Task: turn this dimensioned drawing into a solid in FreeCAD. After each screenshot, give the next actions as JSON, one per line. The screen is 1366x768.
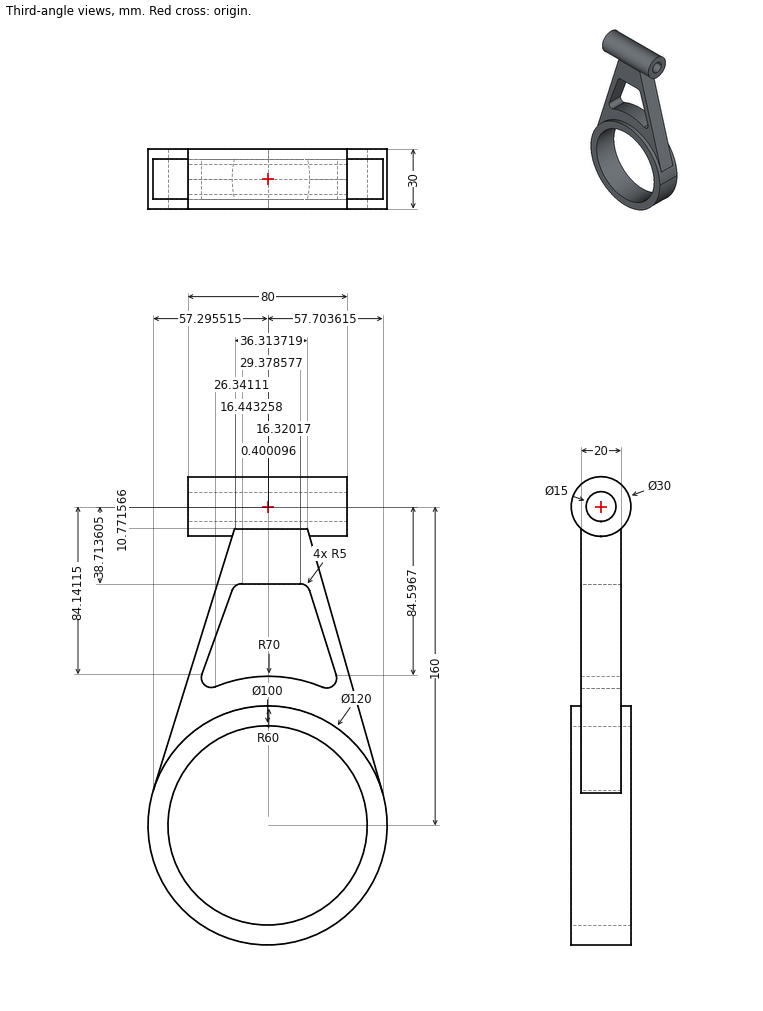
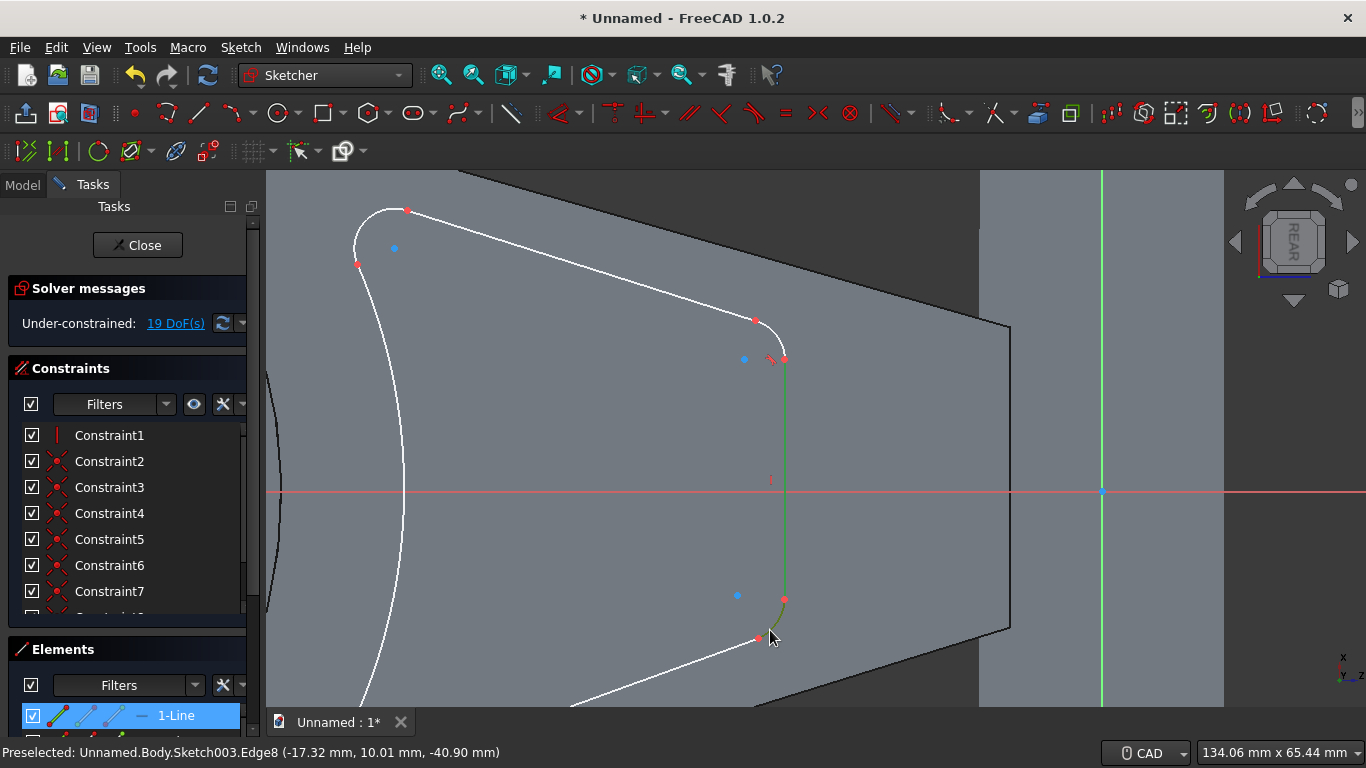
{"action": "left_click", "coordinate": [754, 114]}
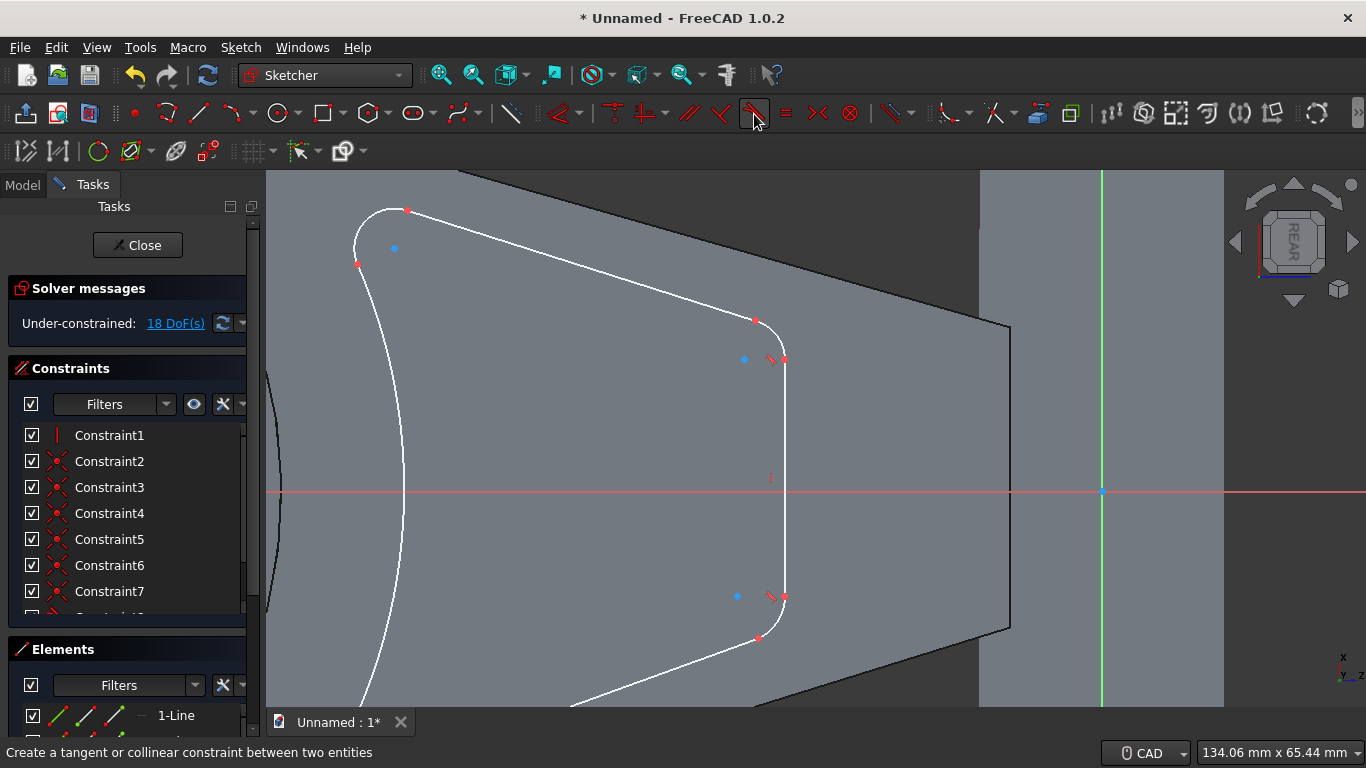
{"action": "left_click", "coordinate": [651, 288]}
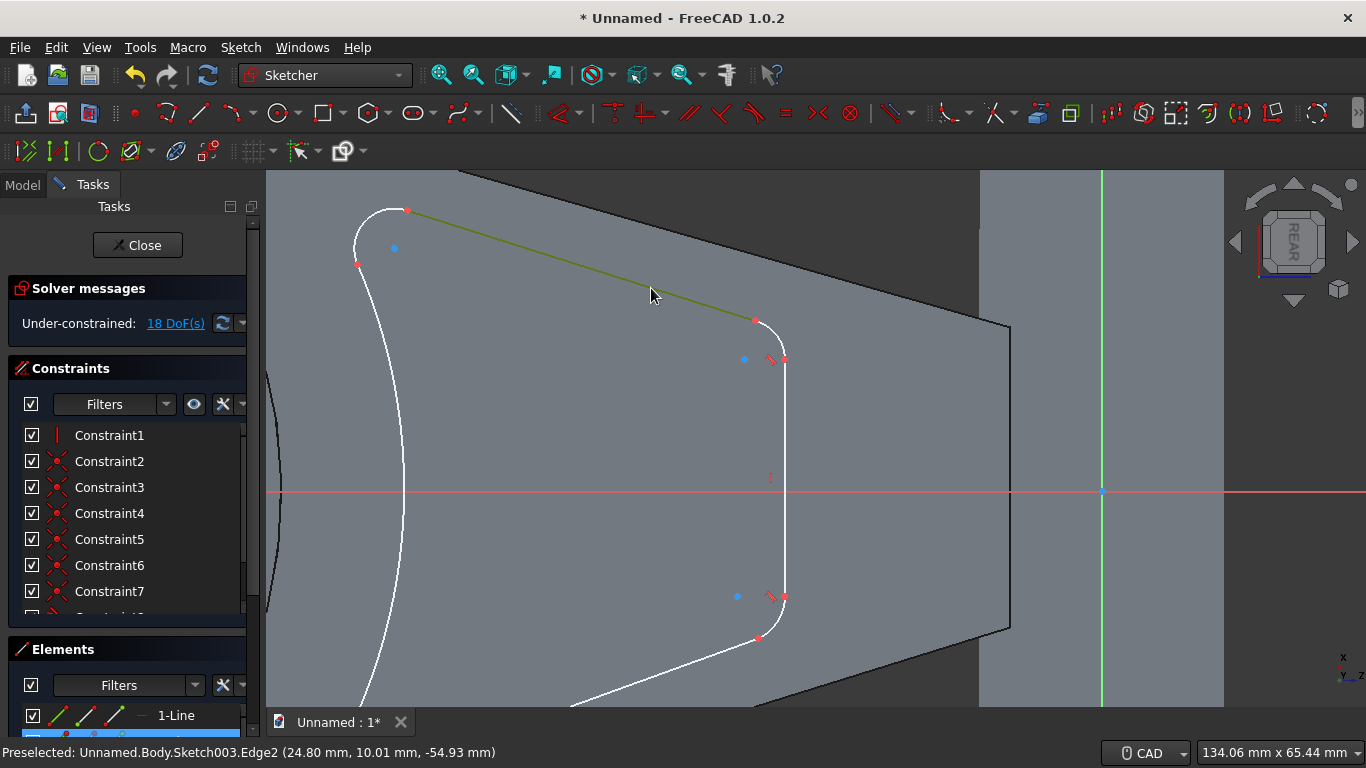
{"action": "left_click", "coordinate": [782, 344]}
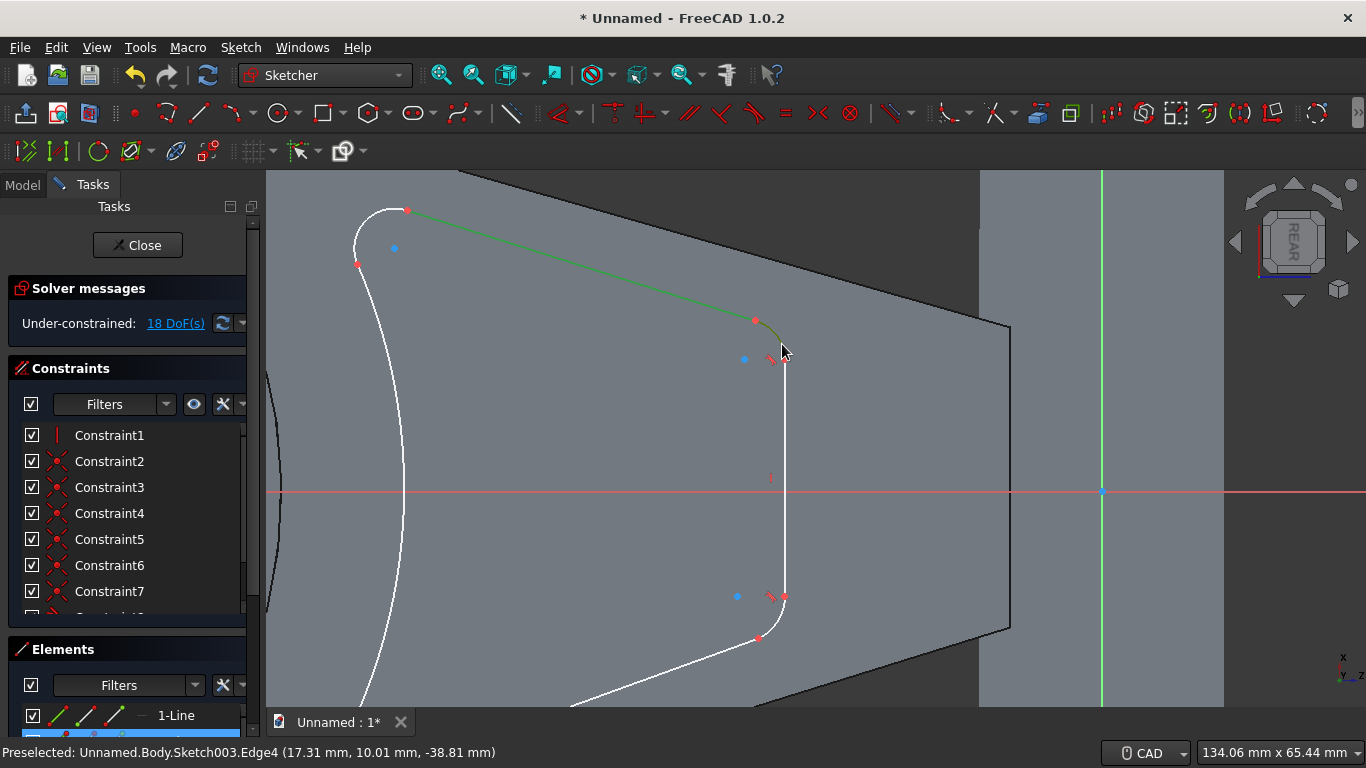
{"action": "left_click", "coordinate": [754, 114]}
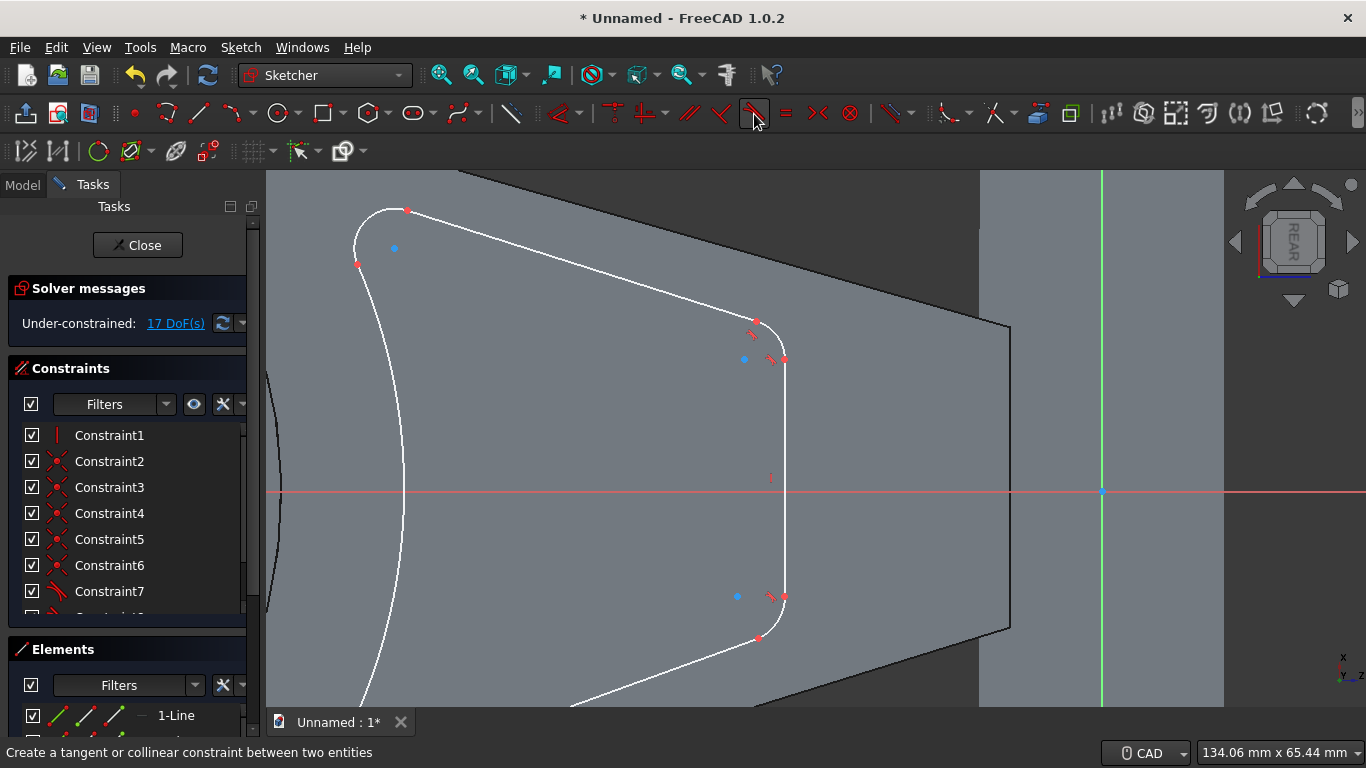
{"action": "left_click", "coordinate": [652, 288]}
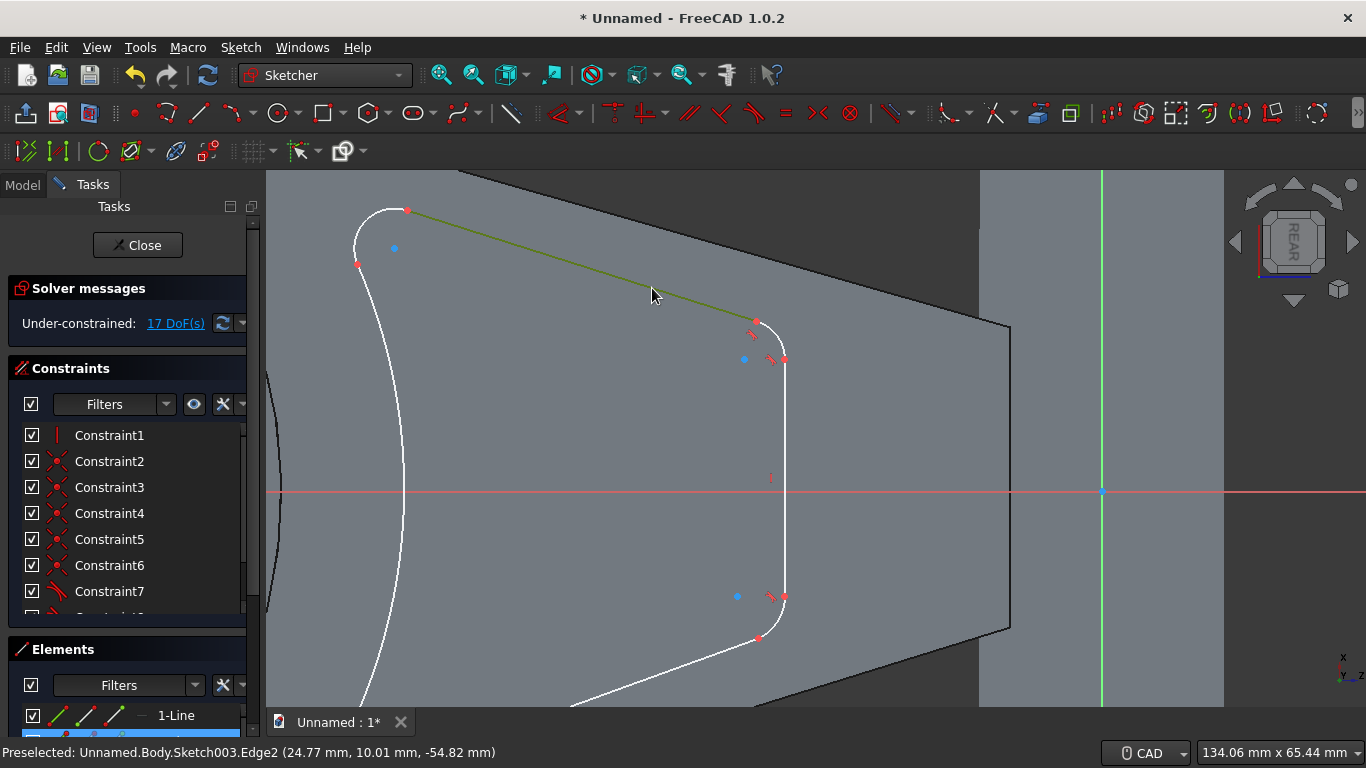
{"action": "left_click", "coordinate": [380, 211]}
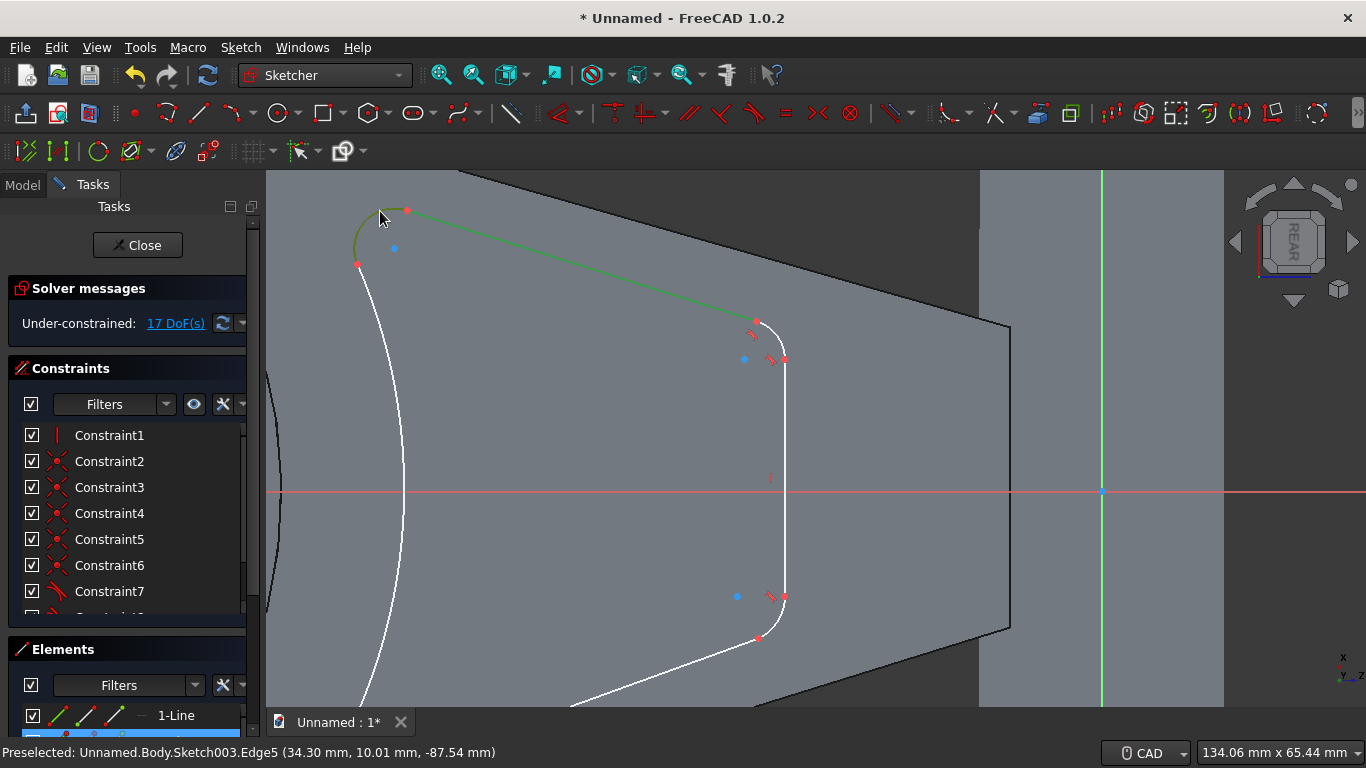
{"action": "left_click", "coordinate": [754, 114]}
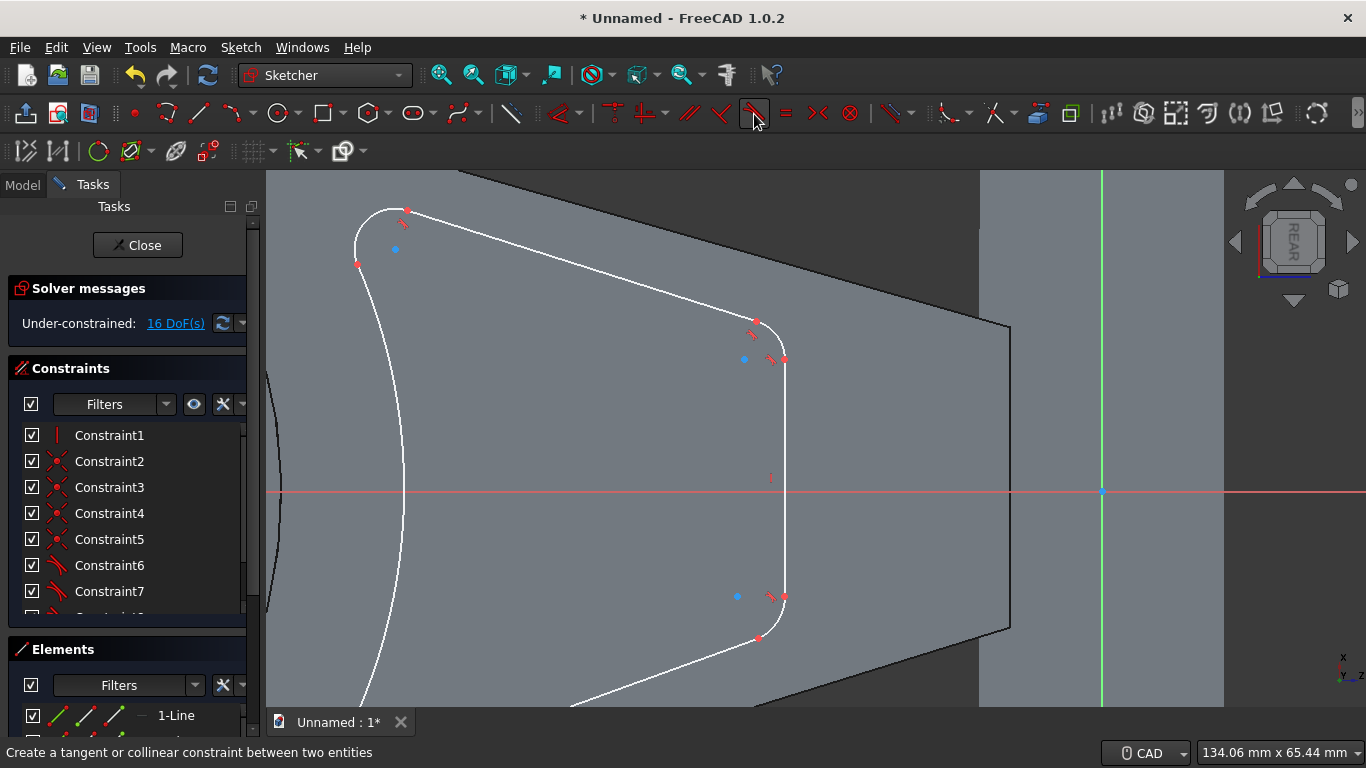
{"action": "left_click", "coordinate": [654, 676]}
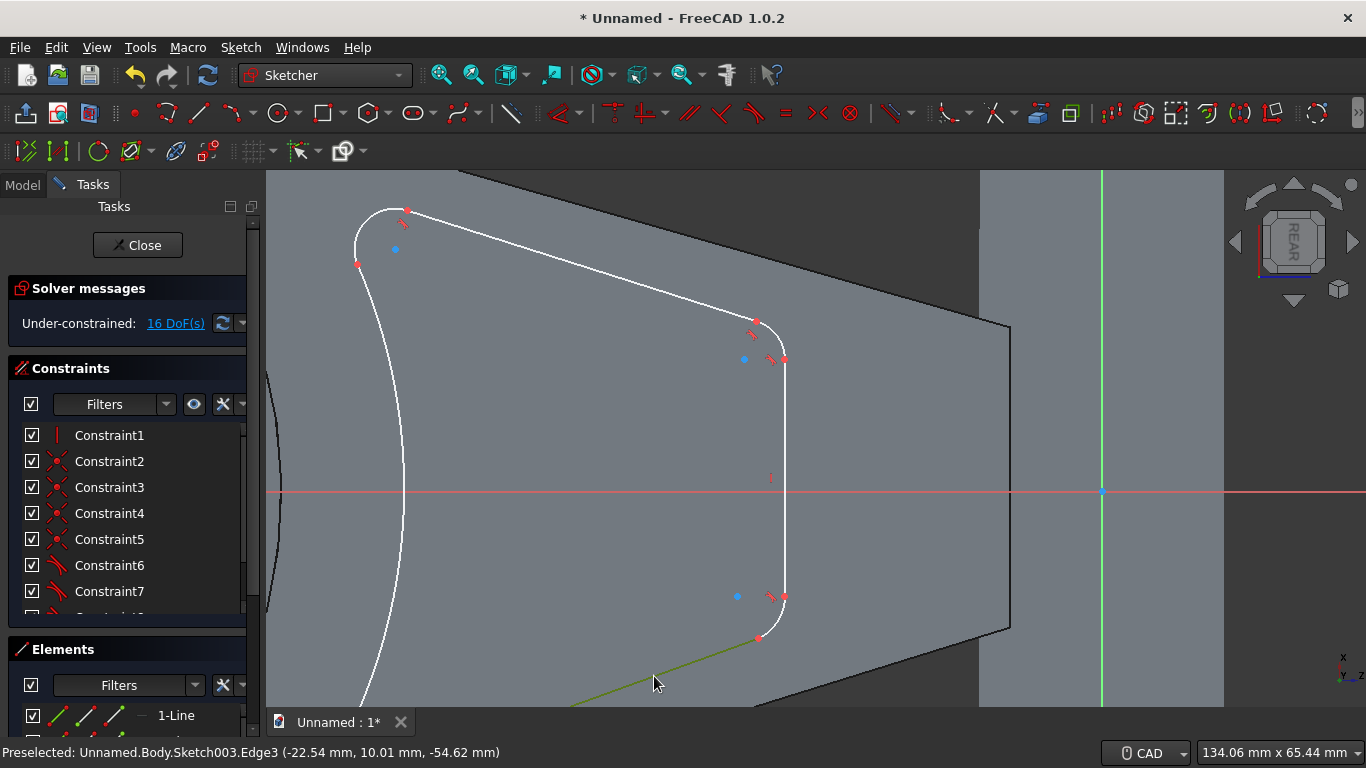
{"action": "scroll", "coordinate": [783, 343], "scroll_direction": "down", "scroll_amount": 2}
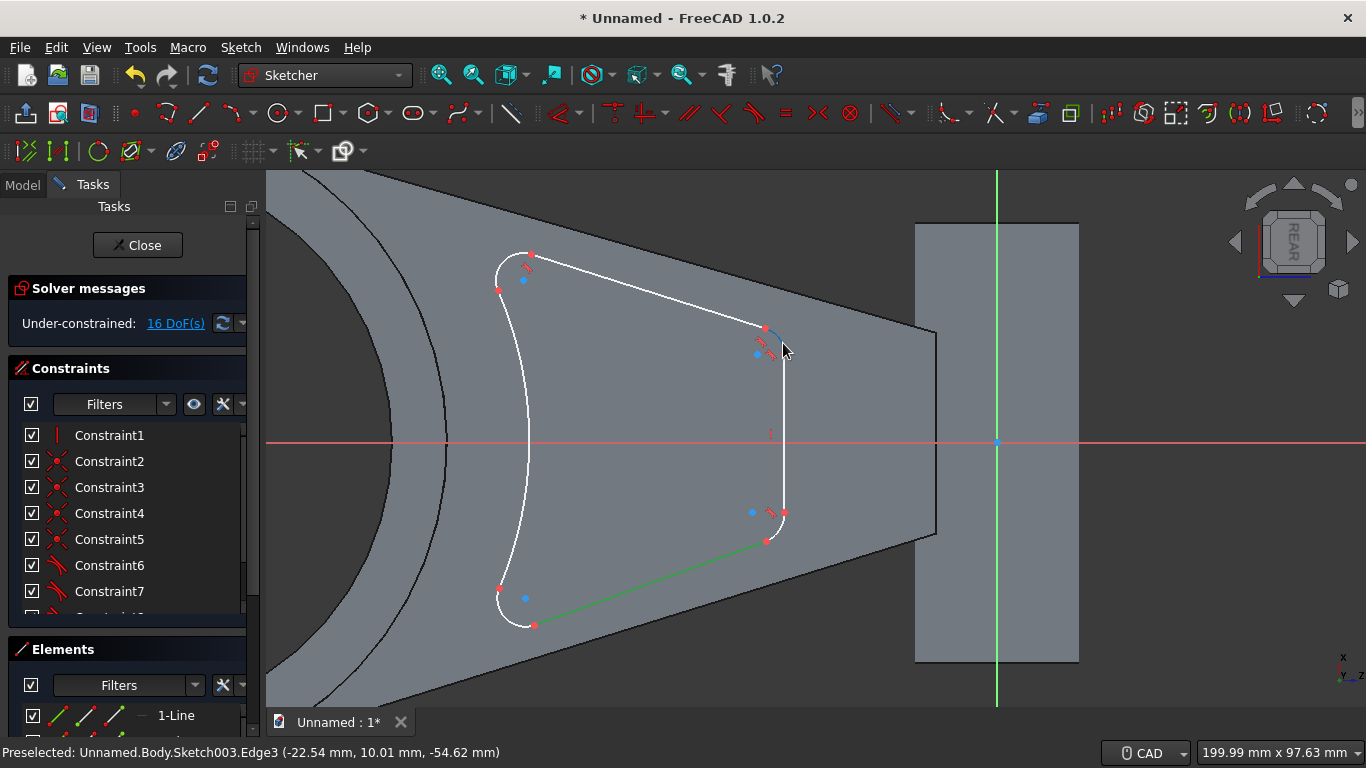
{"action": "left_click", "coordinate": [499, 607]}